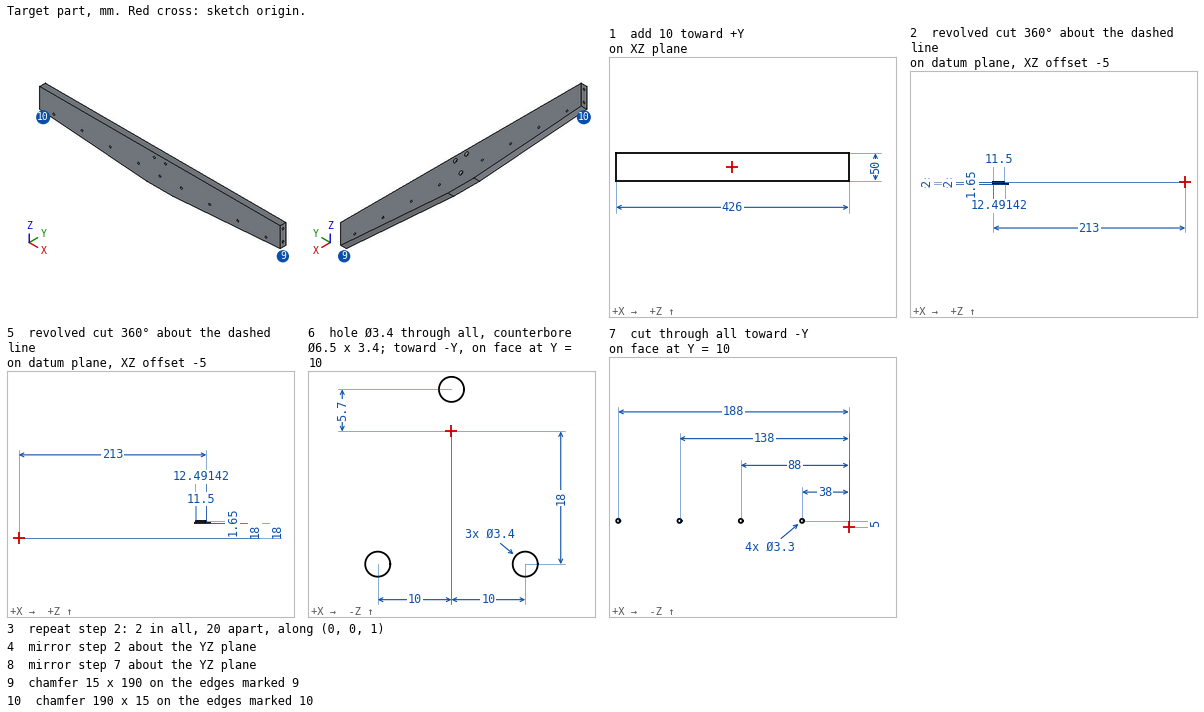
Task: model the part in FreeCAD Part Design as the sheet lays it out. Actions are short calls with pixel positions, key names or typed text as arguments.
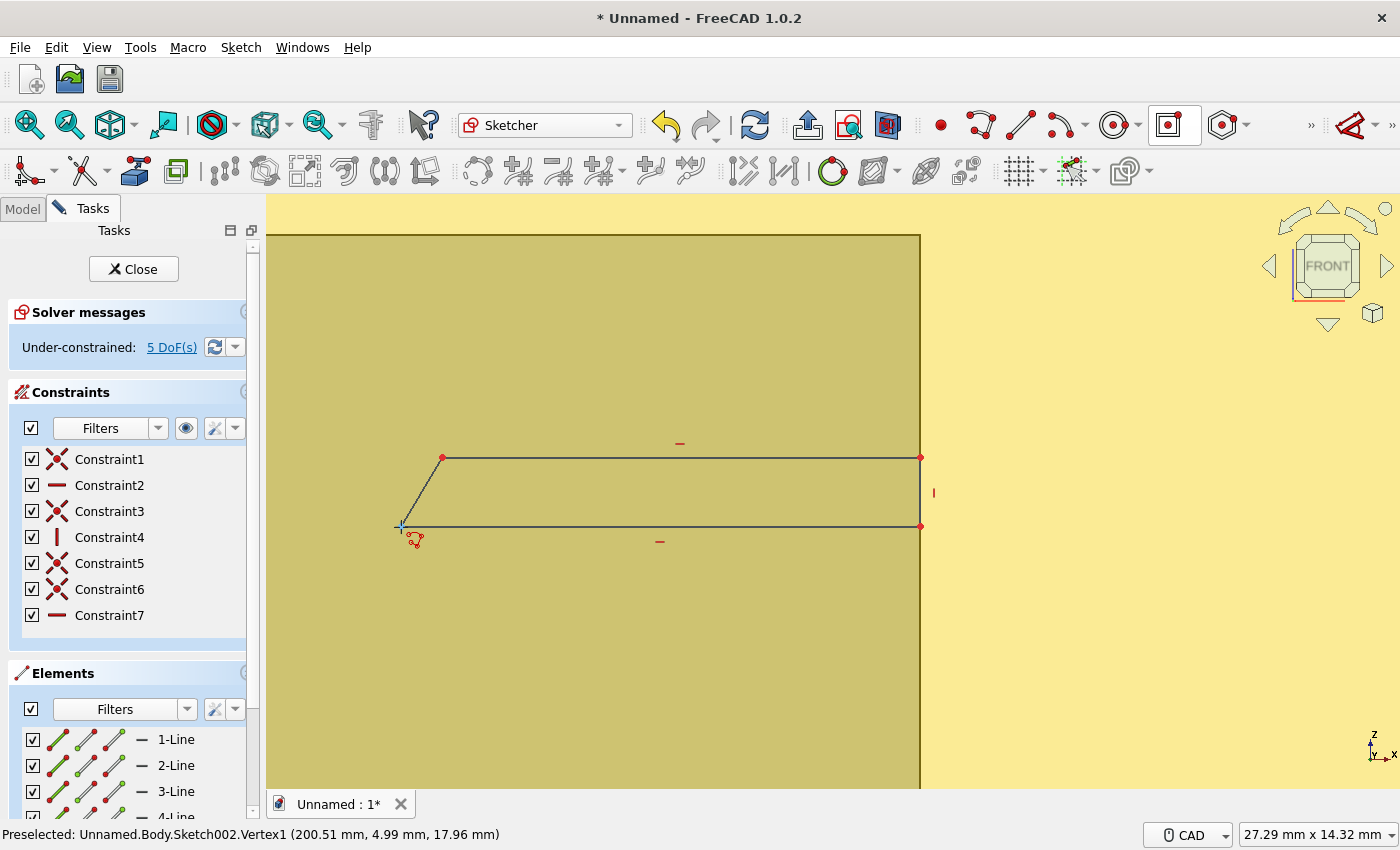
click(1022, 126)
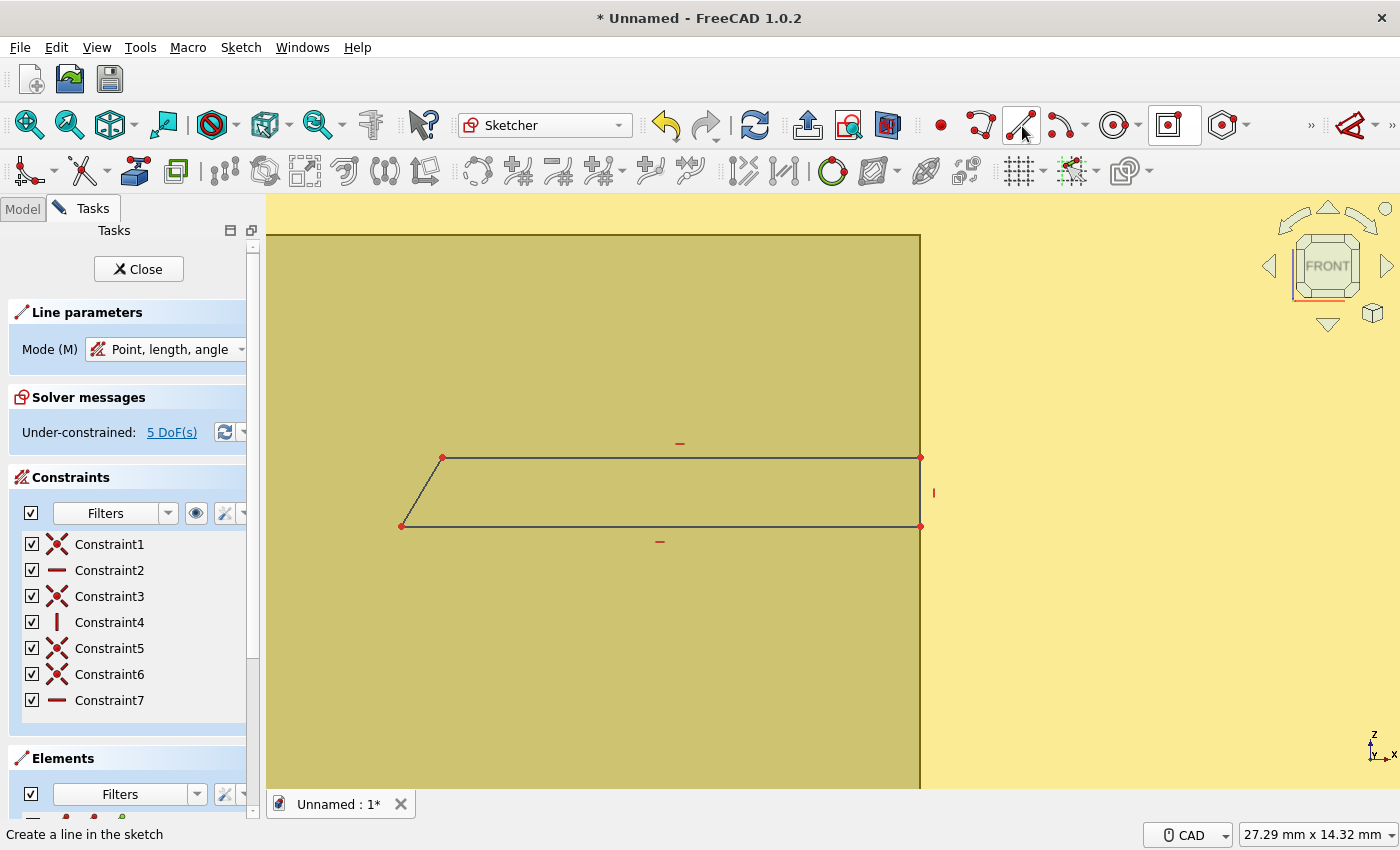
click(972, 526)
click(1128, 526)
key(Escape)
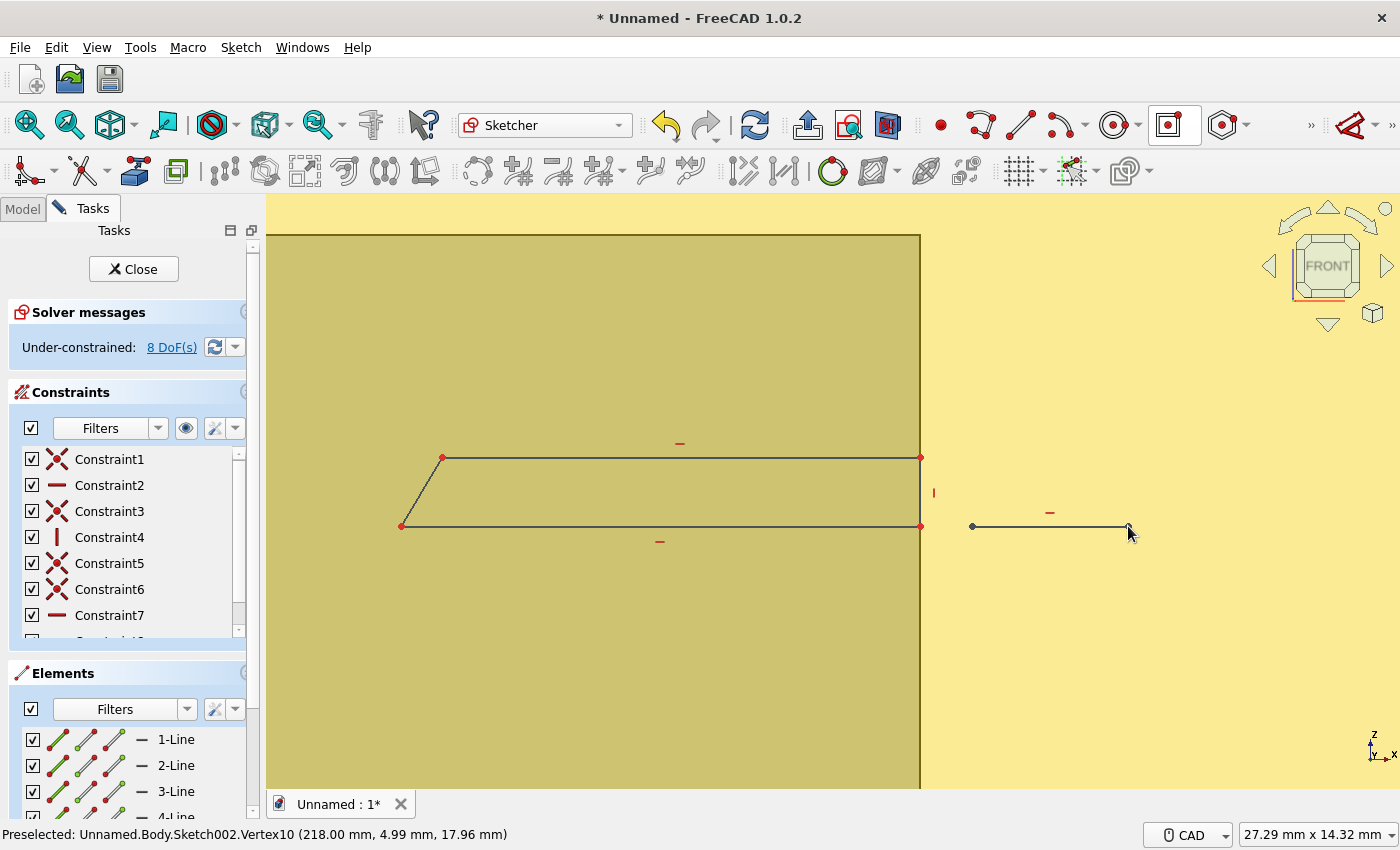
click(1019, 527)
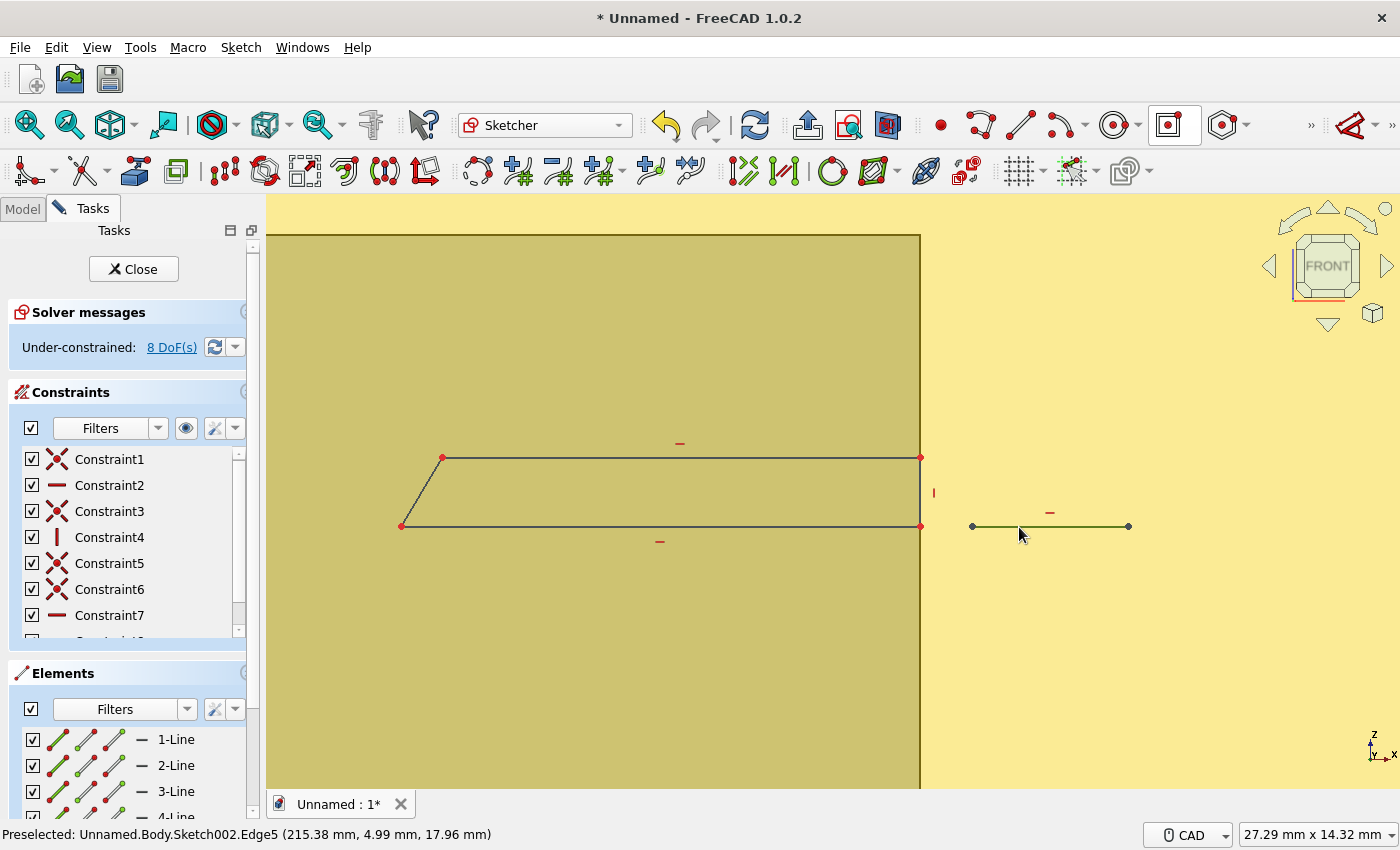
key(g)
key(n)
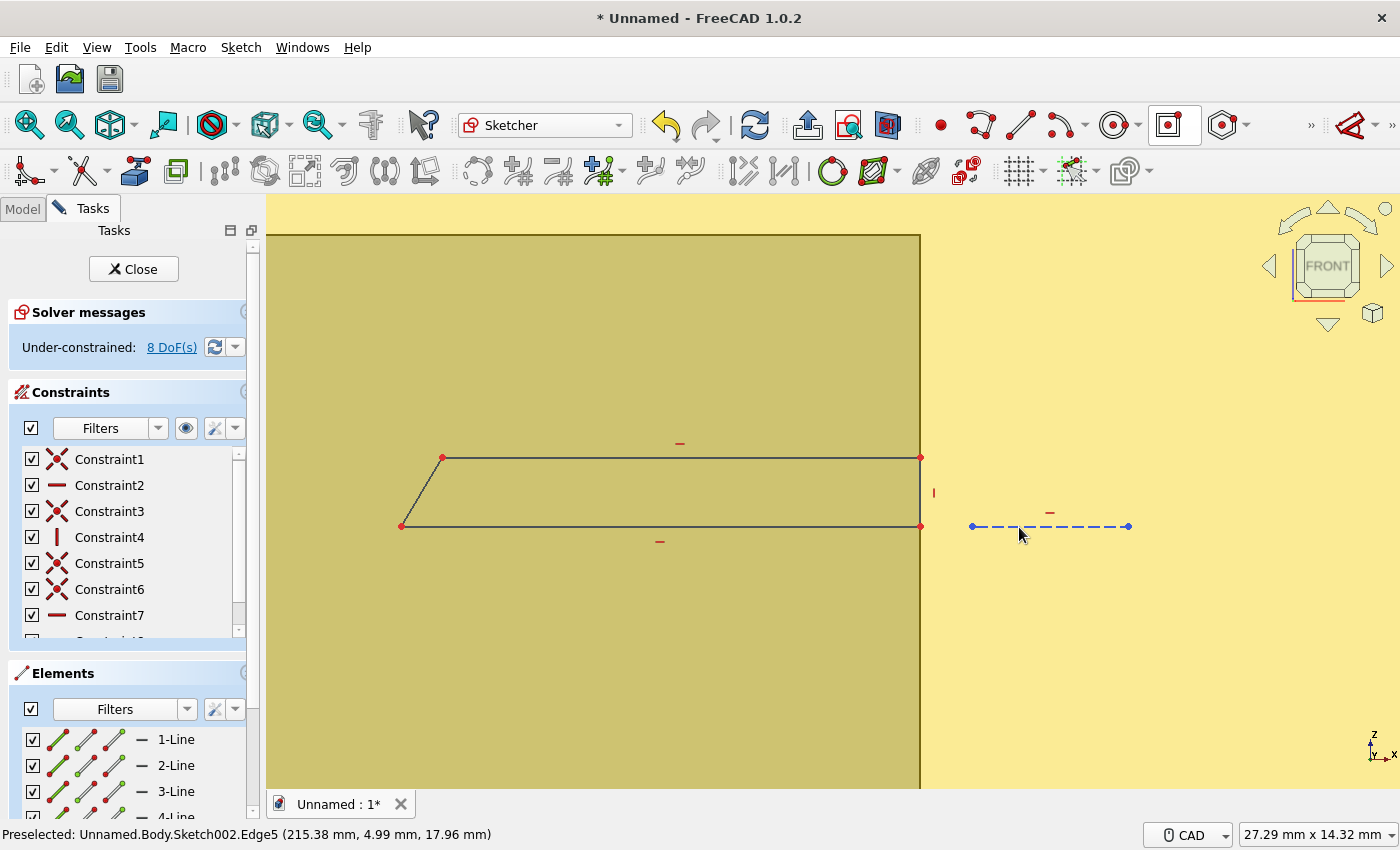
click(1350, 126)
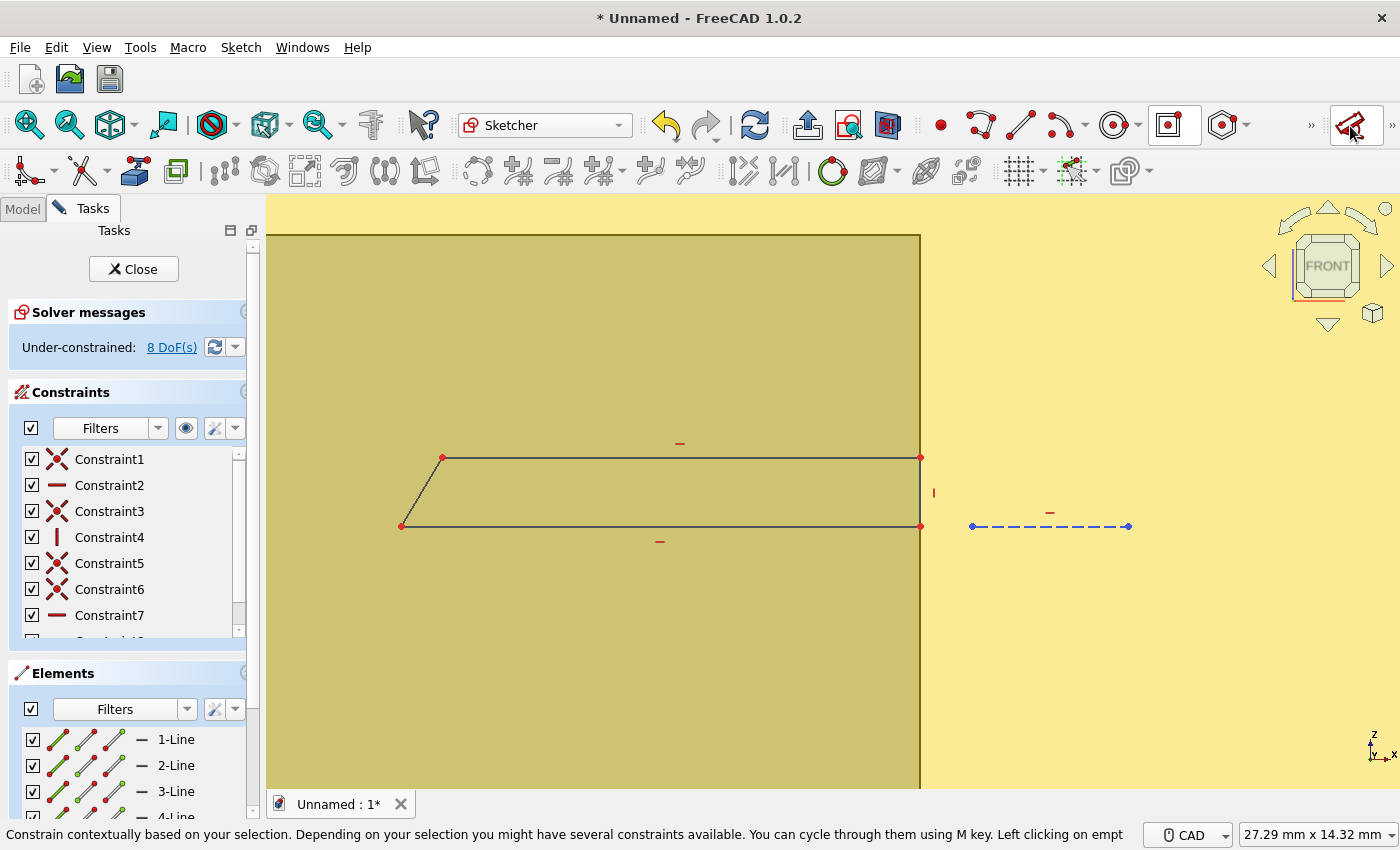
click(401, 527)
click(435, 644)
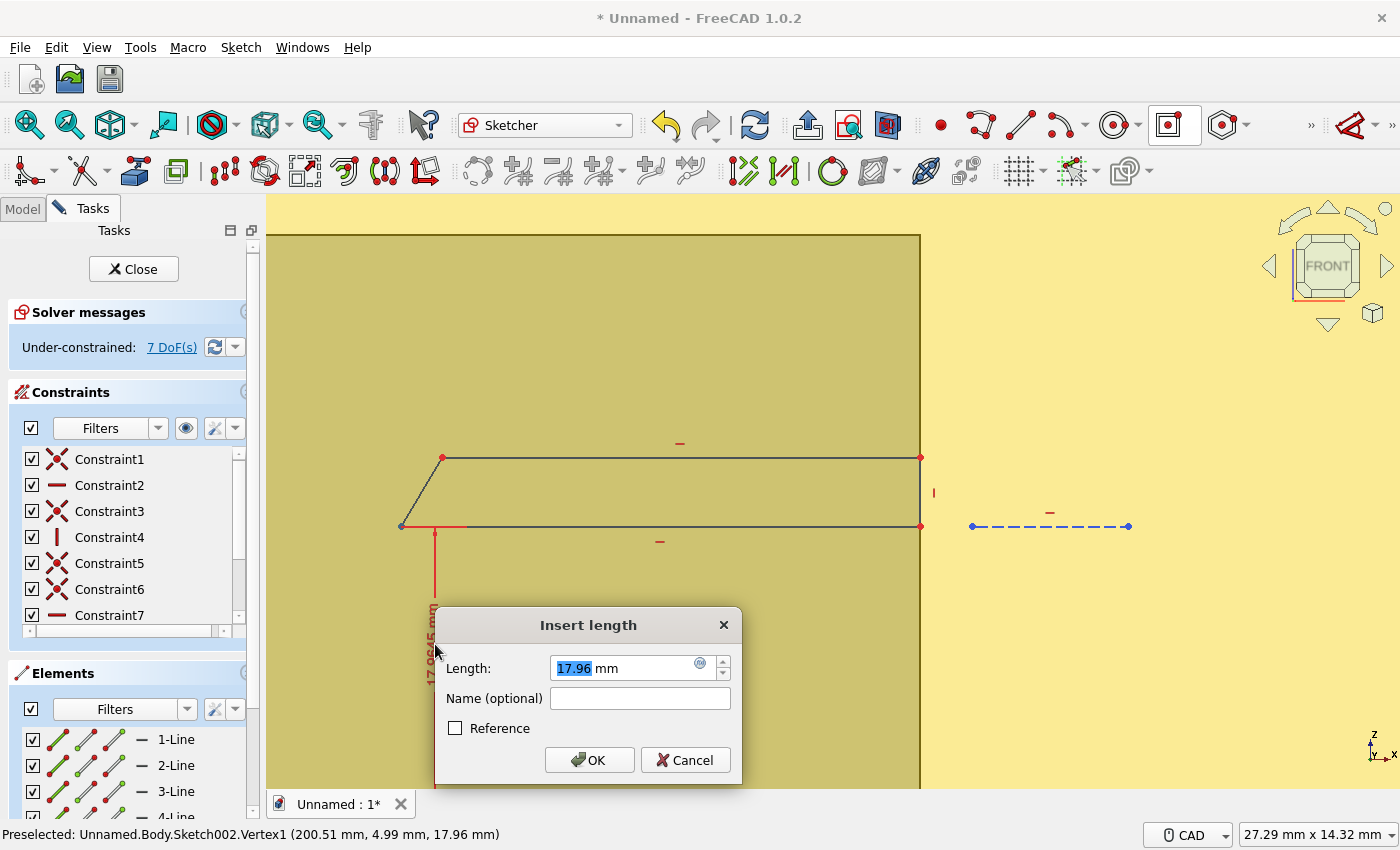
text(18)
key(Return)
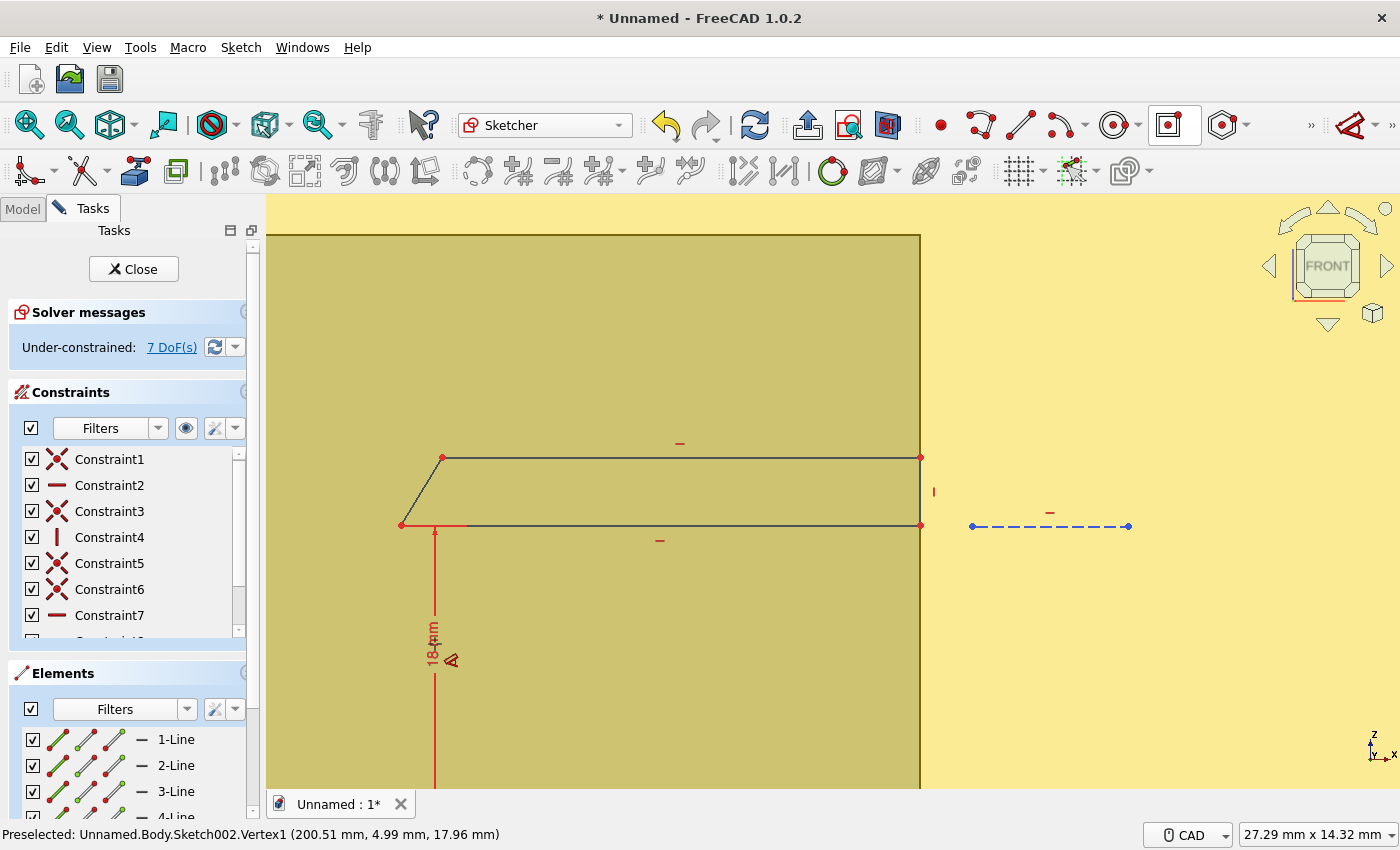
click(972, 527)
click(1006, 644)